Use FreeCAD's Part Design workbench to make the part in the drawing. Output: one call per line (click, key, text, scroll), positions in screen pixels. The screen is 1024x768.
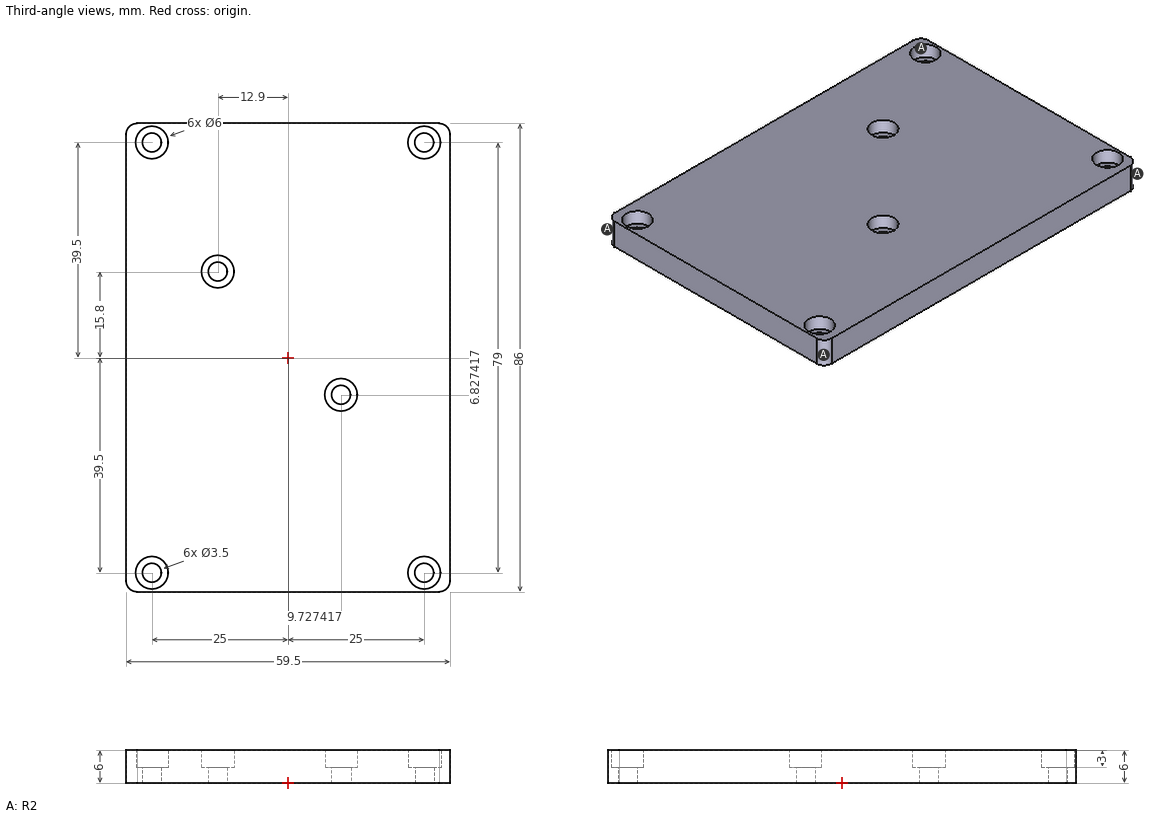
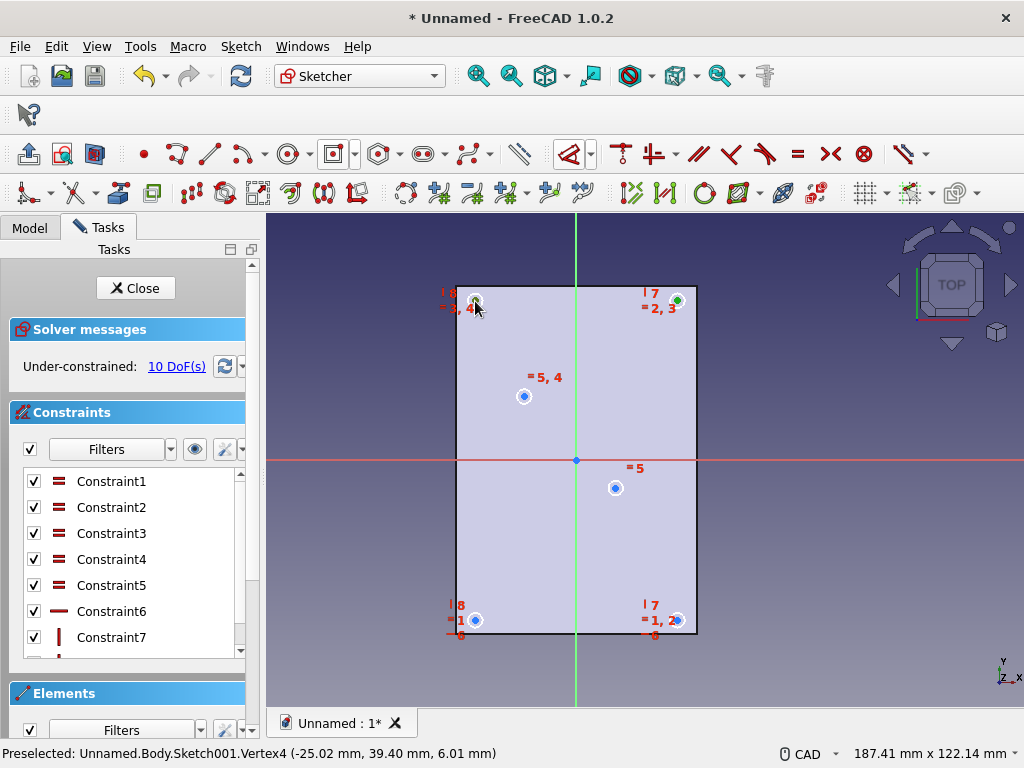
key(h)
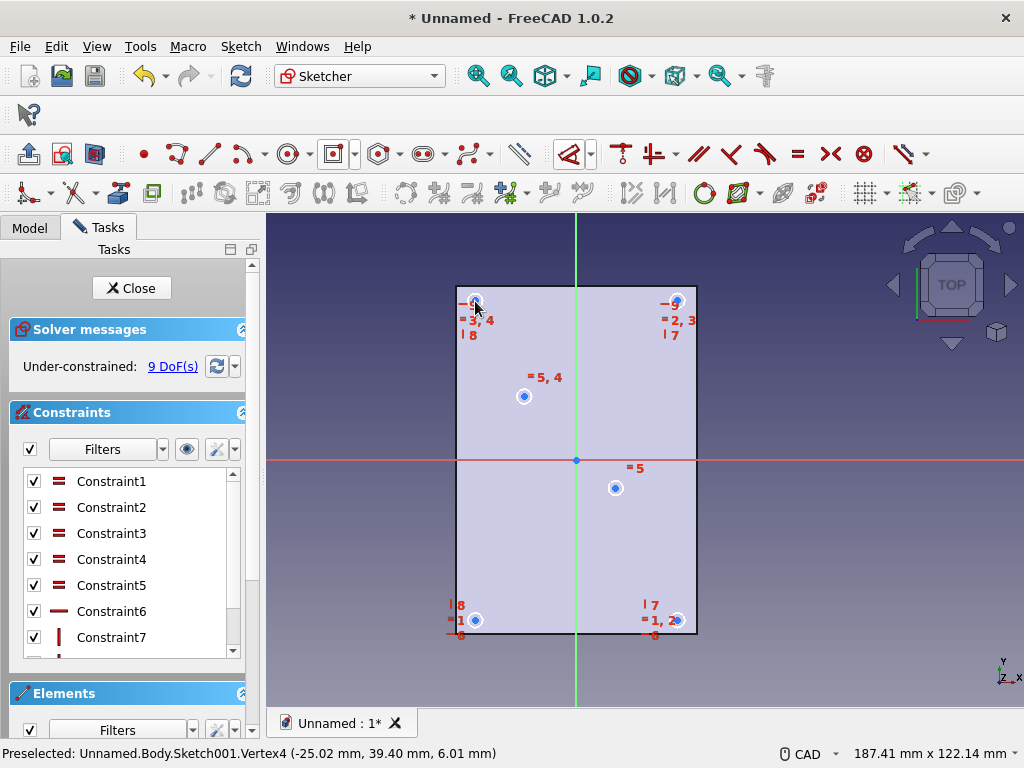
click(568, 154)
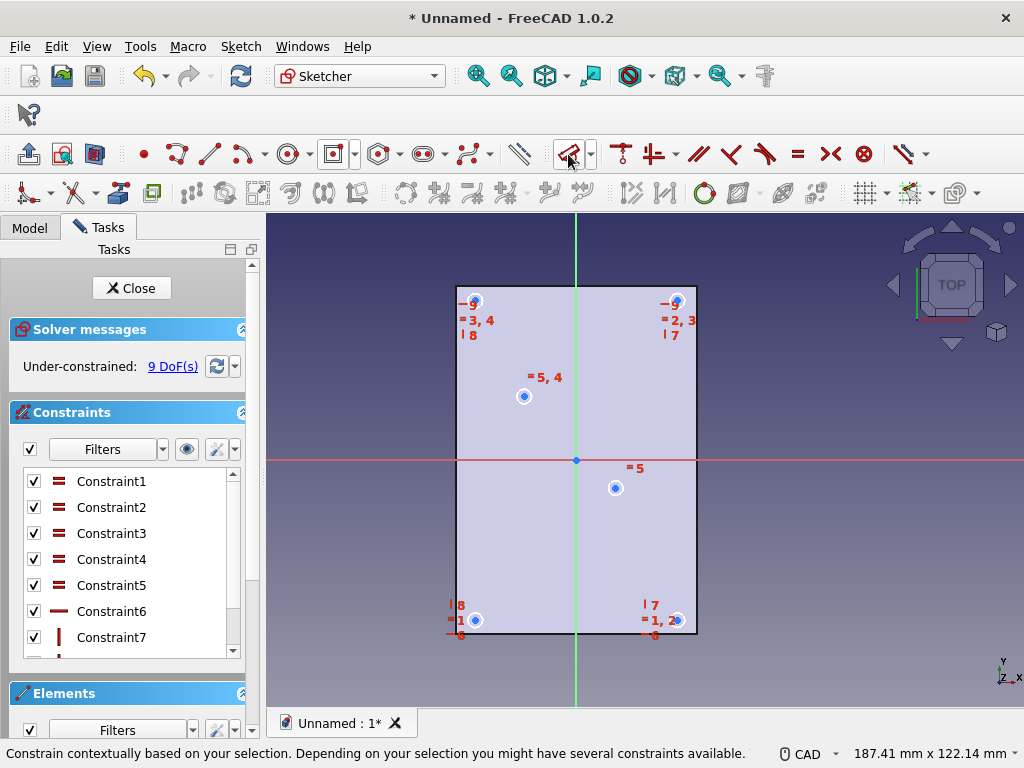
scroll(480, 615, up, 6)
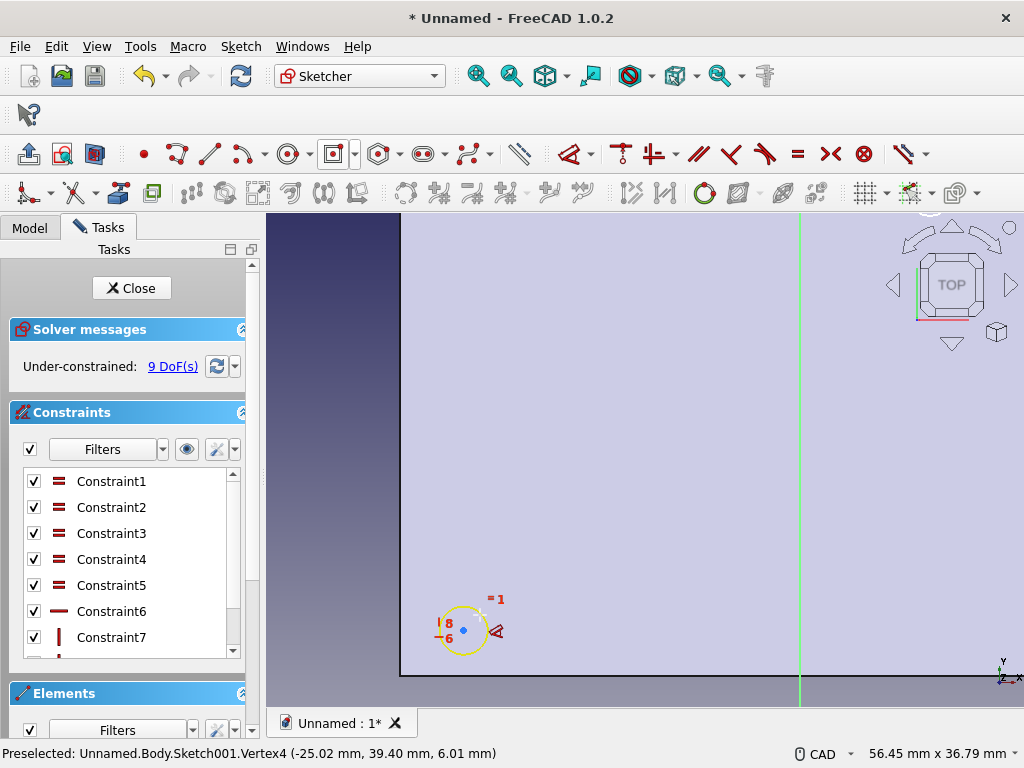
click(481, 614)
click(504, 592)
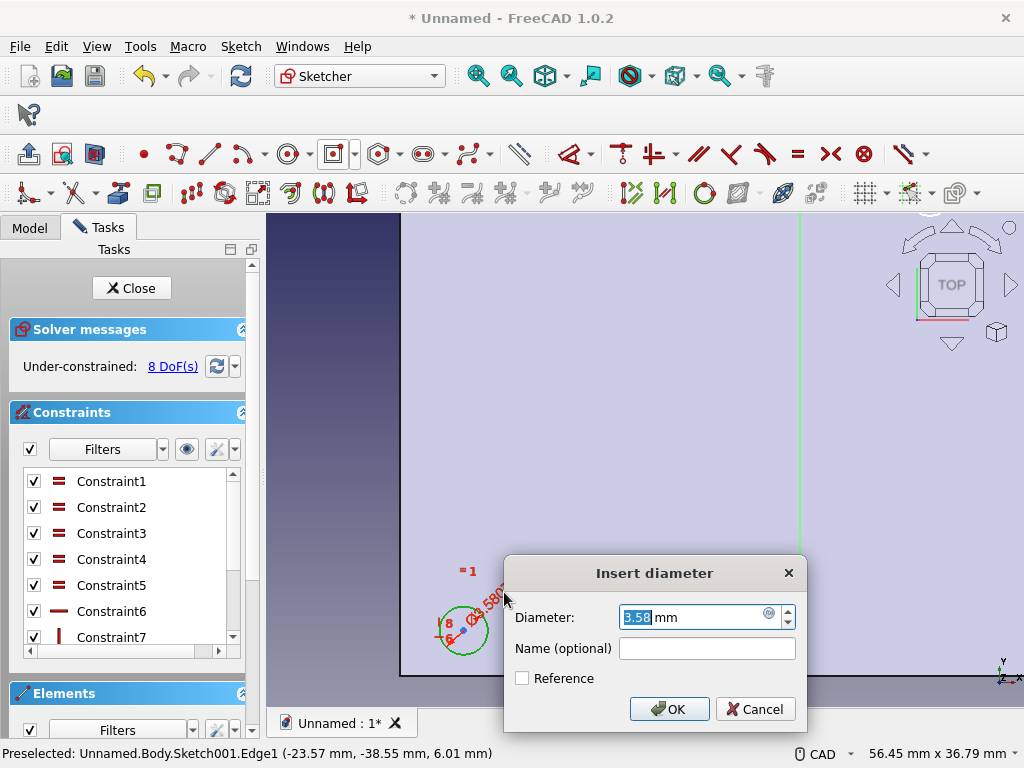
text(3.5)
key(Return)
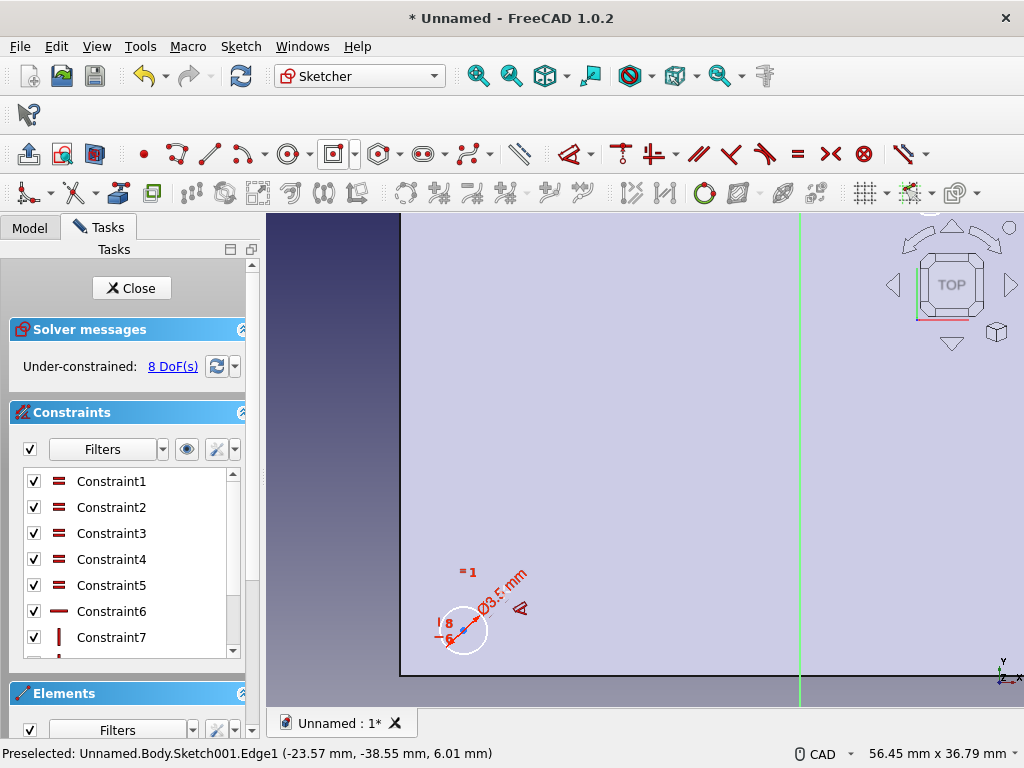
click(464, 631)
click(632, 665)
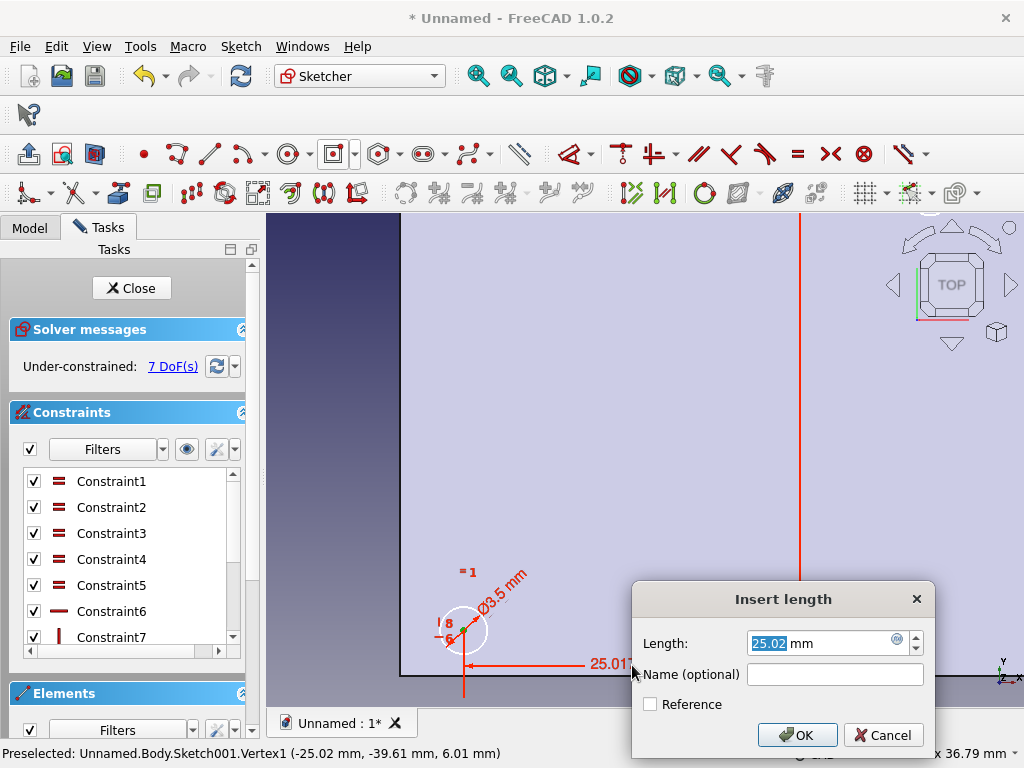
text(25)
key(Return)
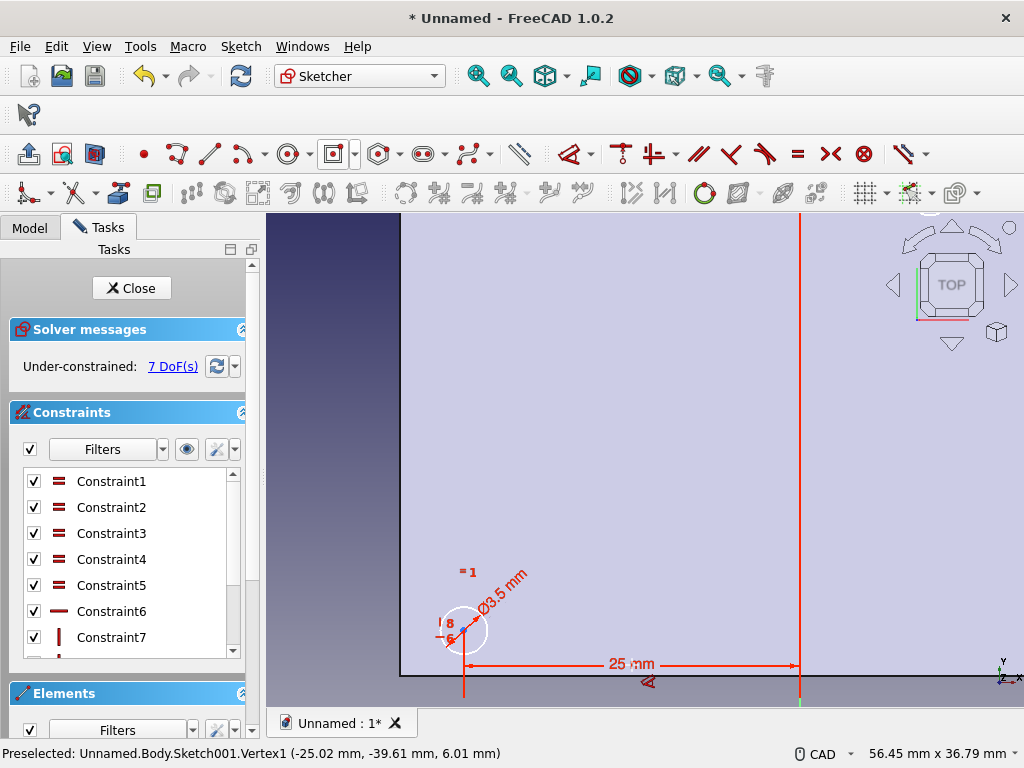
scroll(480, 616, down, 6)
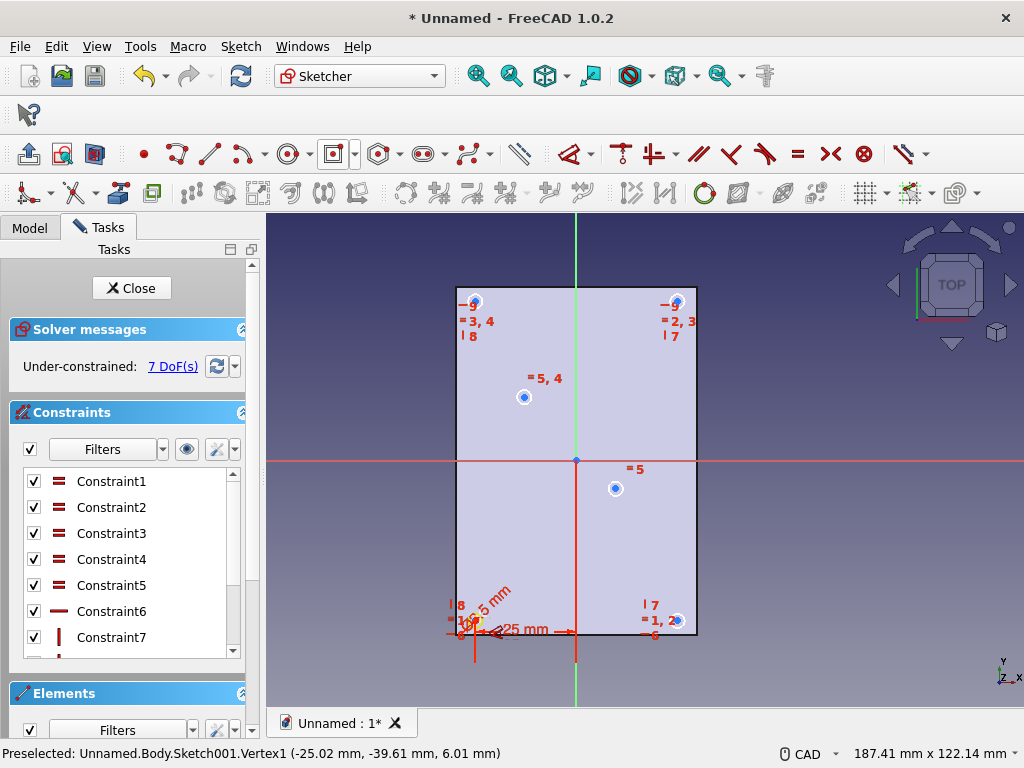
click(677, 621)
click(627, 655)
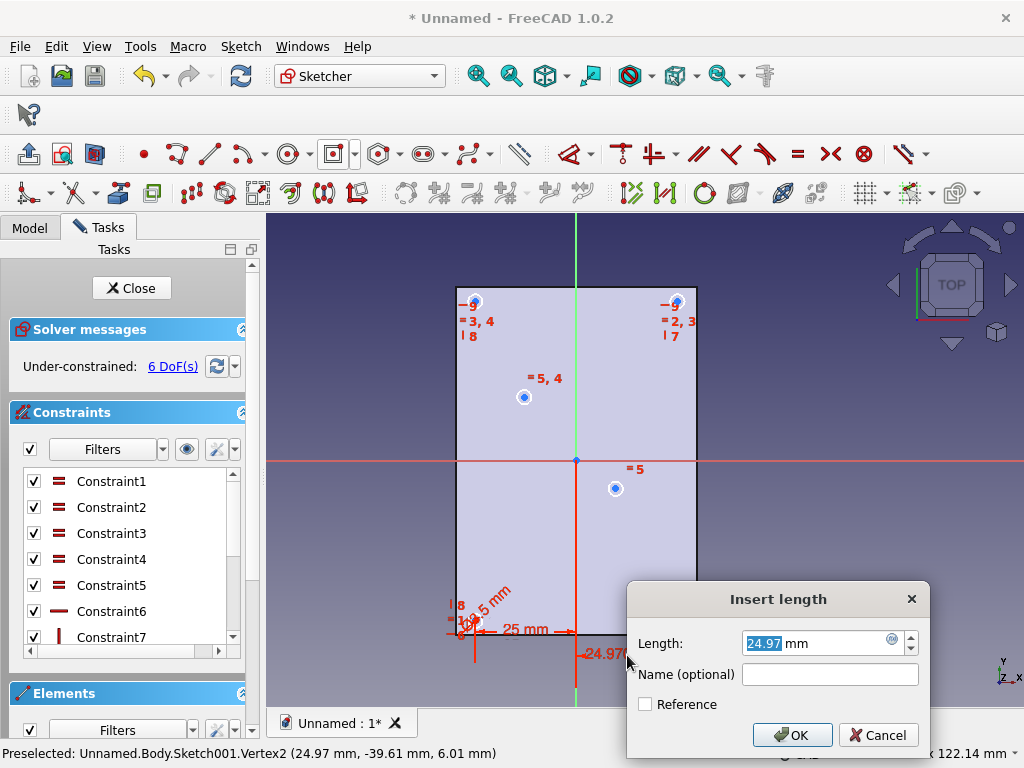
text(25)
key(Return)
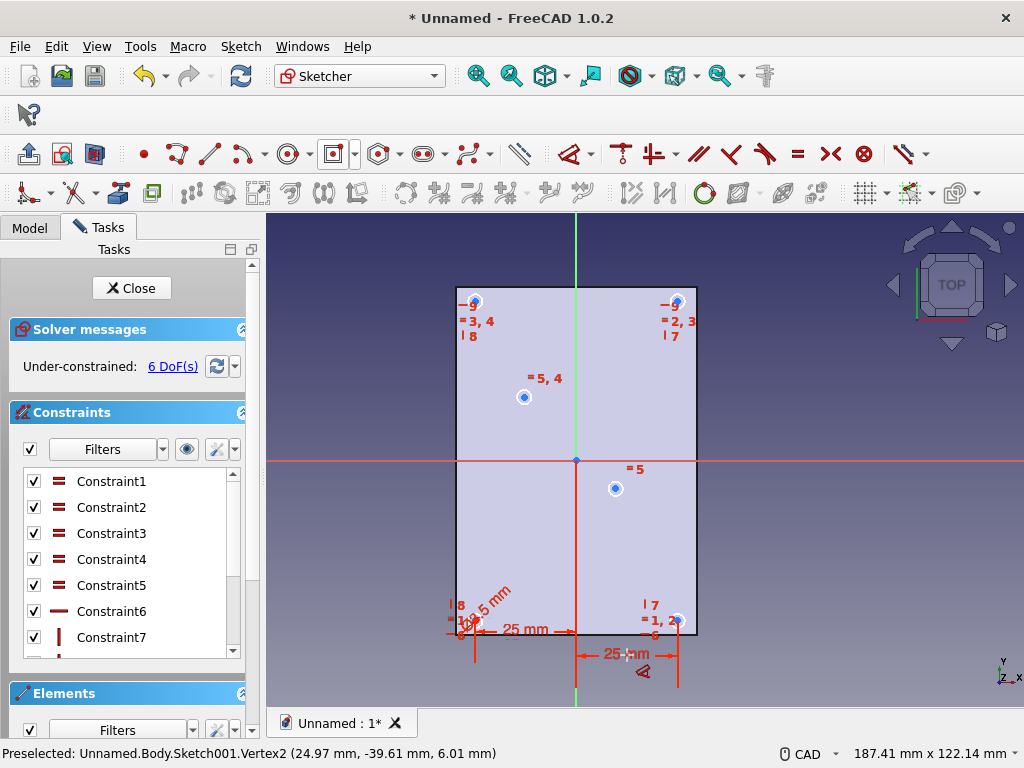
click(678, 621)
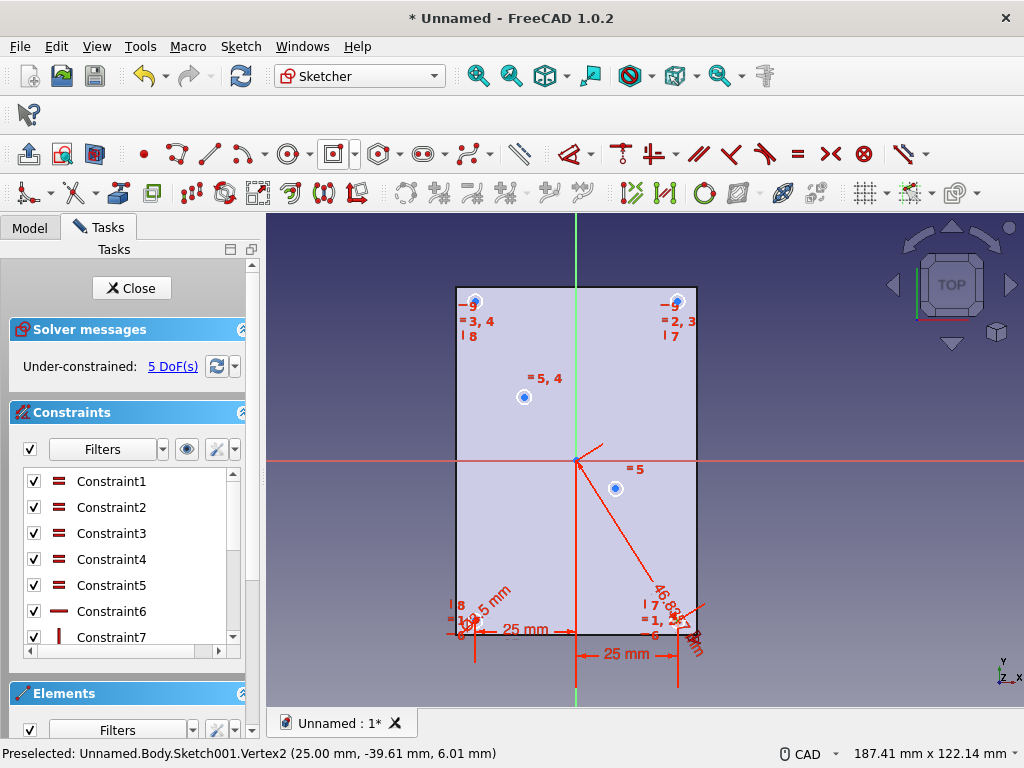
click(678, 301)
click(712, 388)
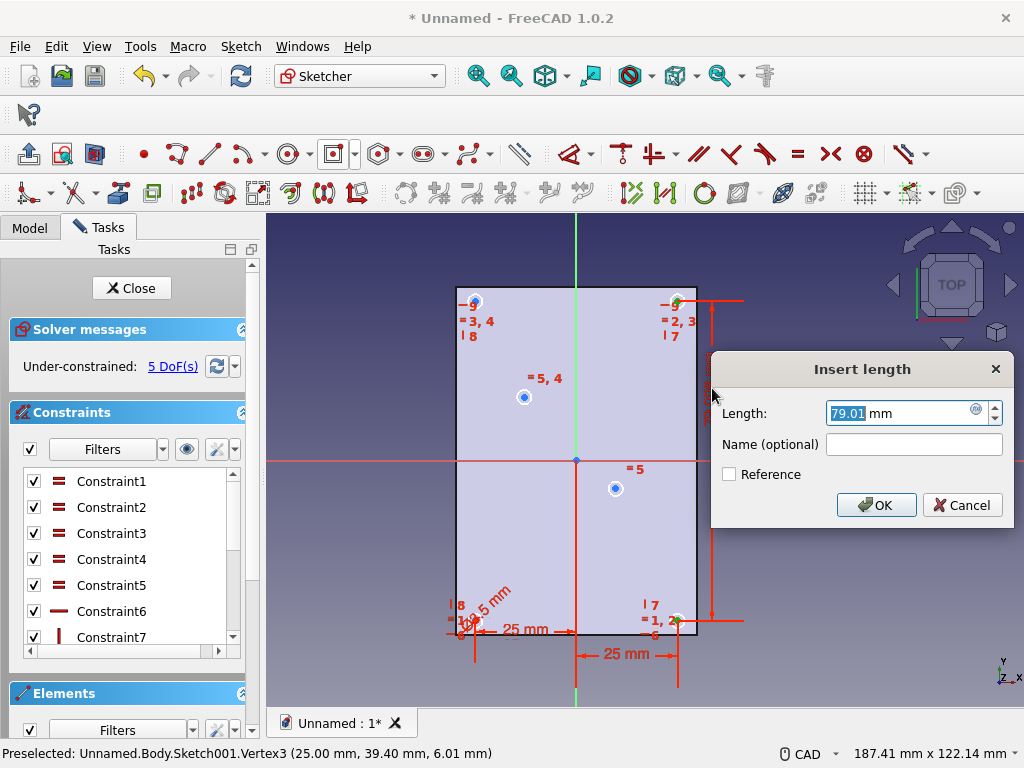
text(79)
key(Return)